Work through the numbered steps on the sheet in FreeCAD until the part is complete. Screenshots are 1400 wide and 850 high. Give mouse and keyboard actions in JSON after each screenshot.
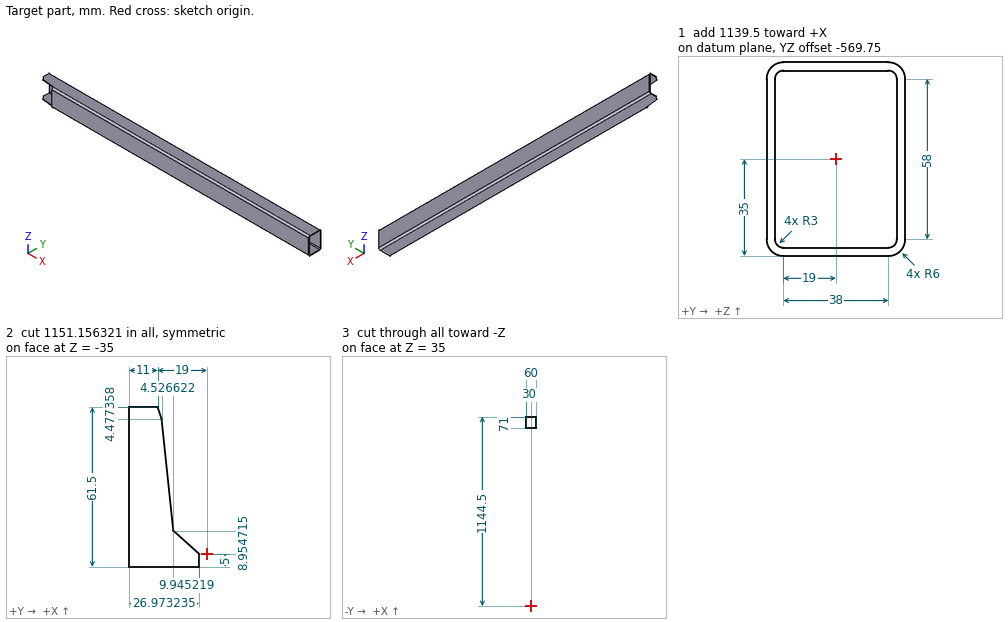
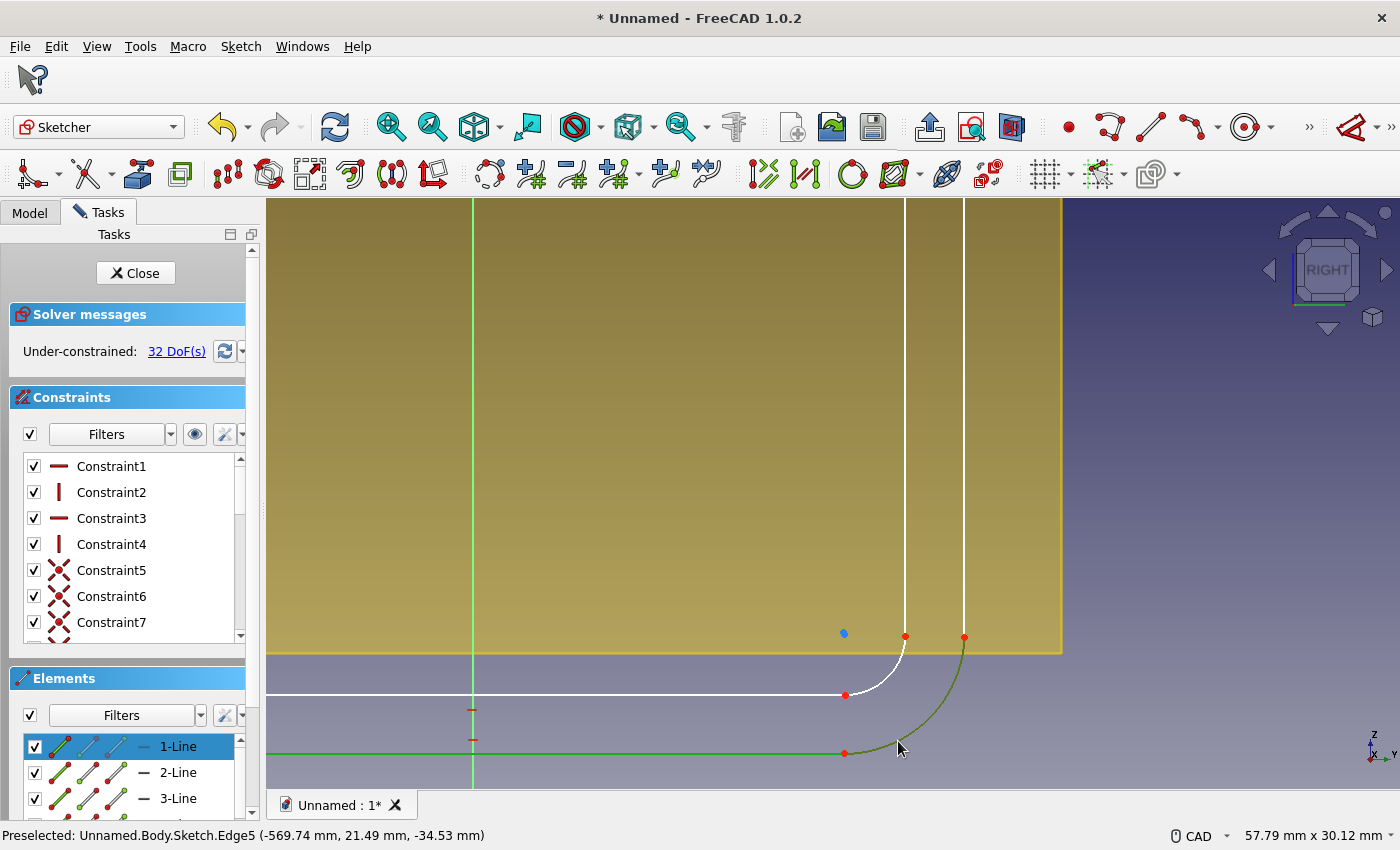
{"action": "key", "text": "t"}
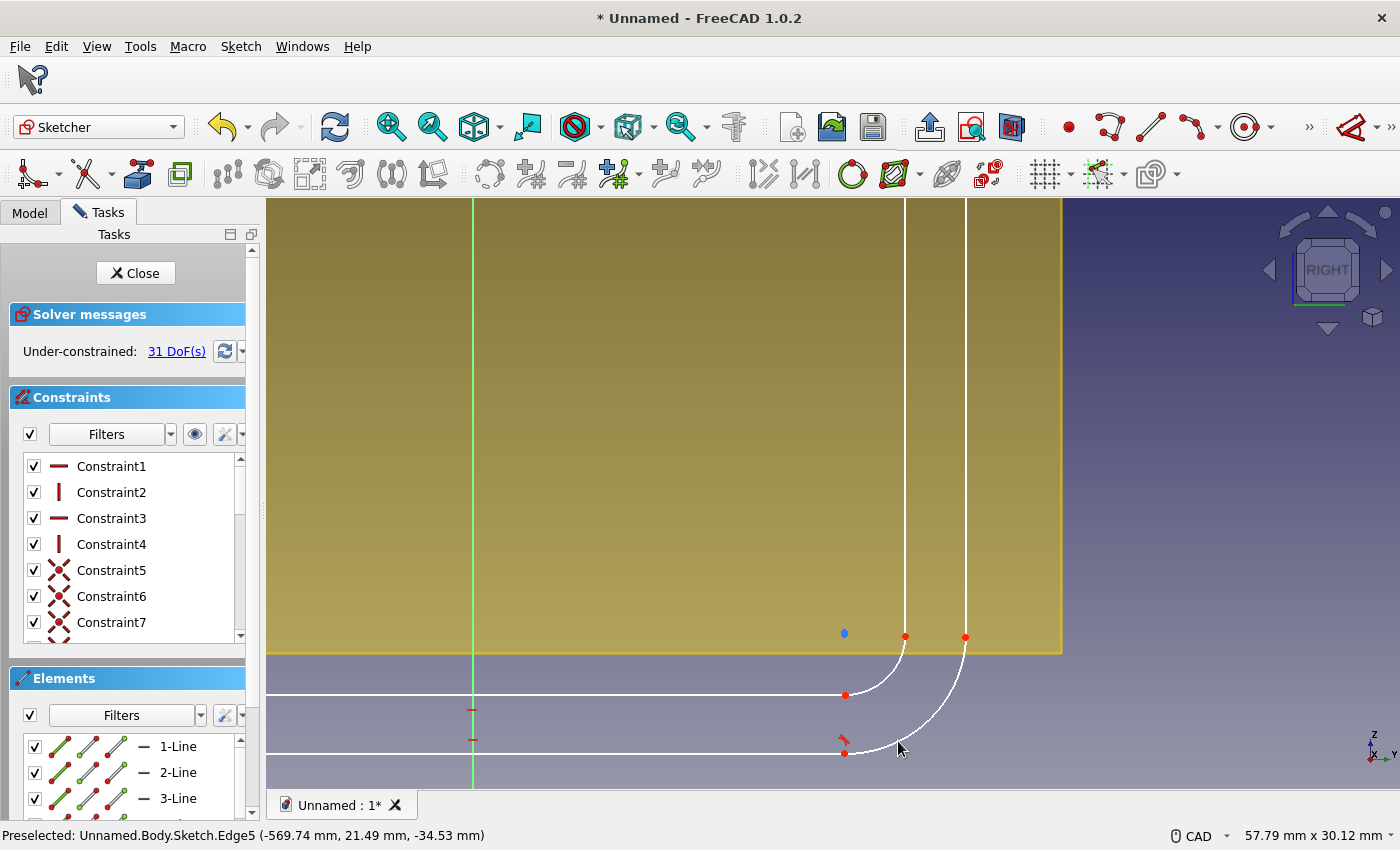
{"action": "left_click", "coordinate": [324, 754]}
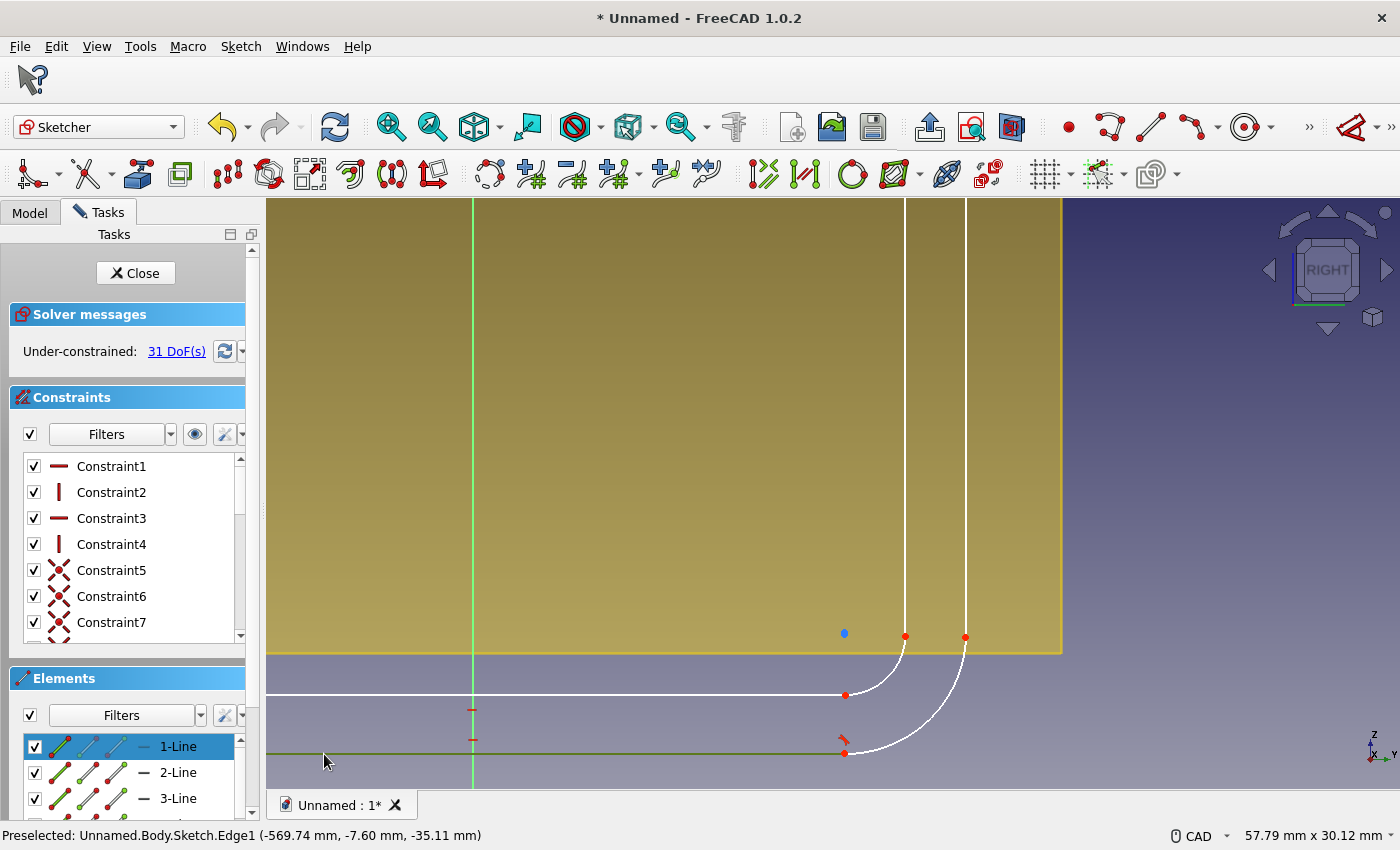
{"action": "scroll", "coordinate": [890, 678], "scroll_direction": "down", "scroll_amount": 6}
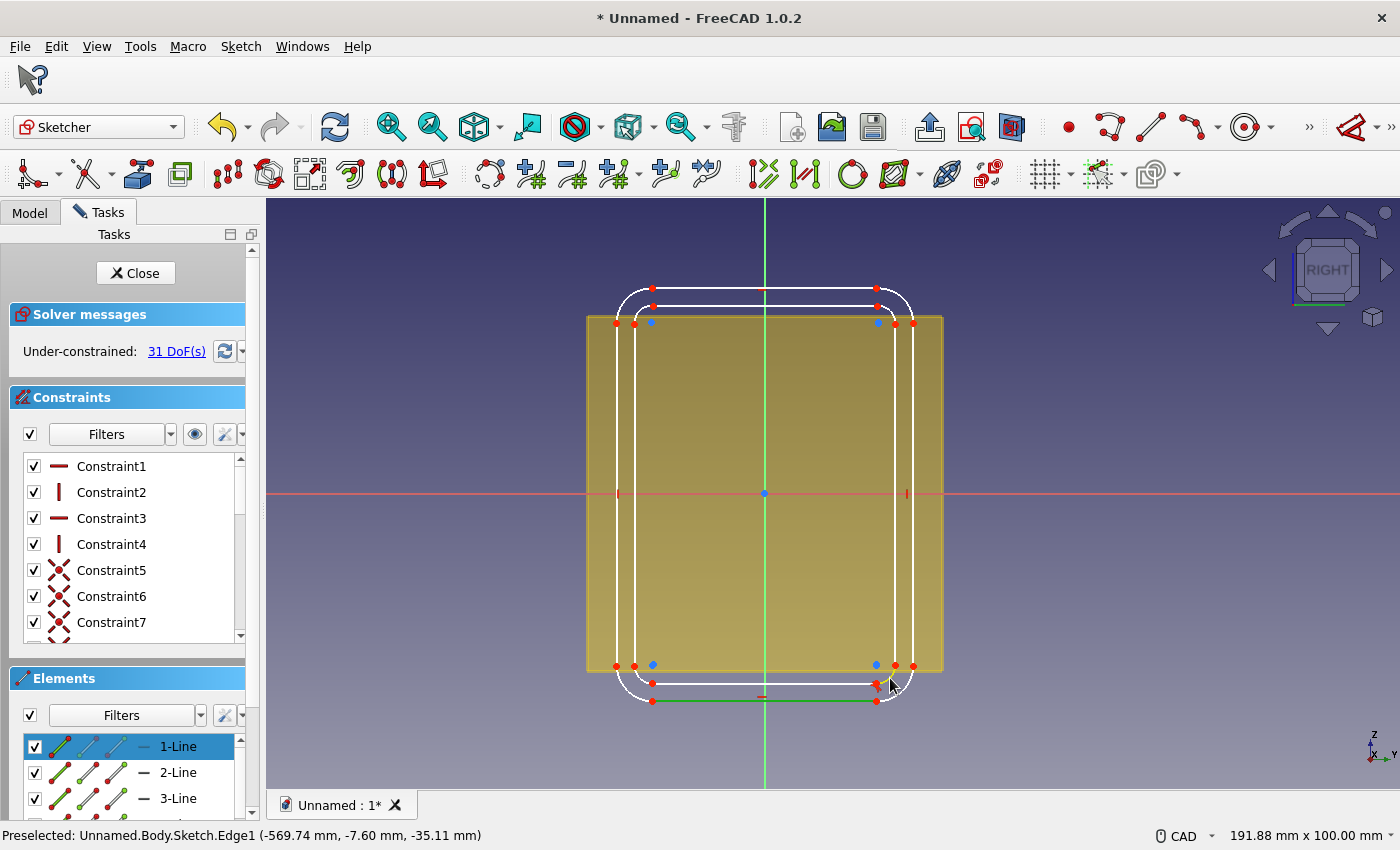
{"action": "left_click", "coordinate": [621, 682]}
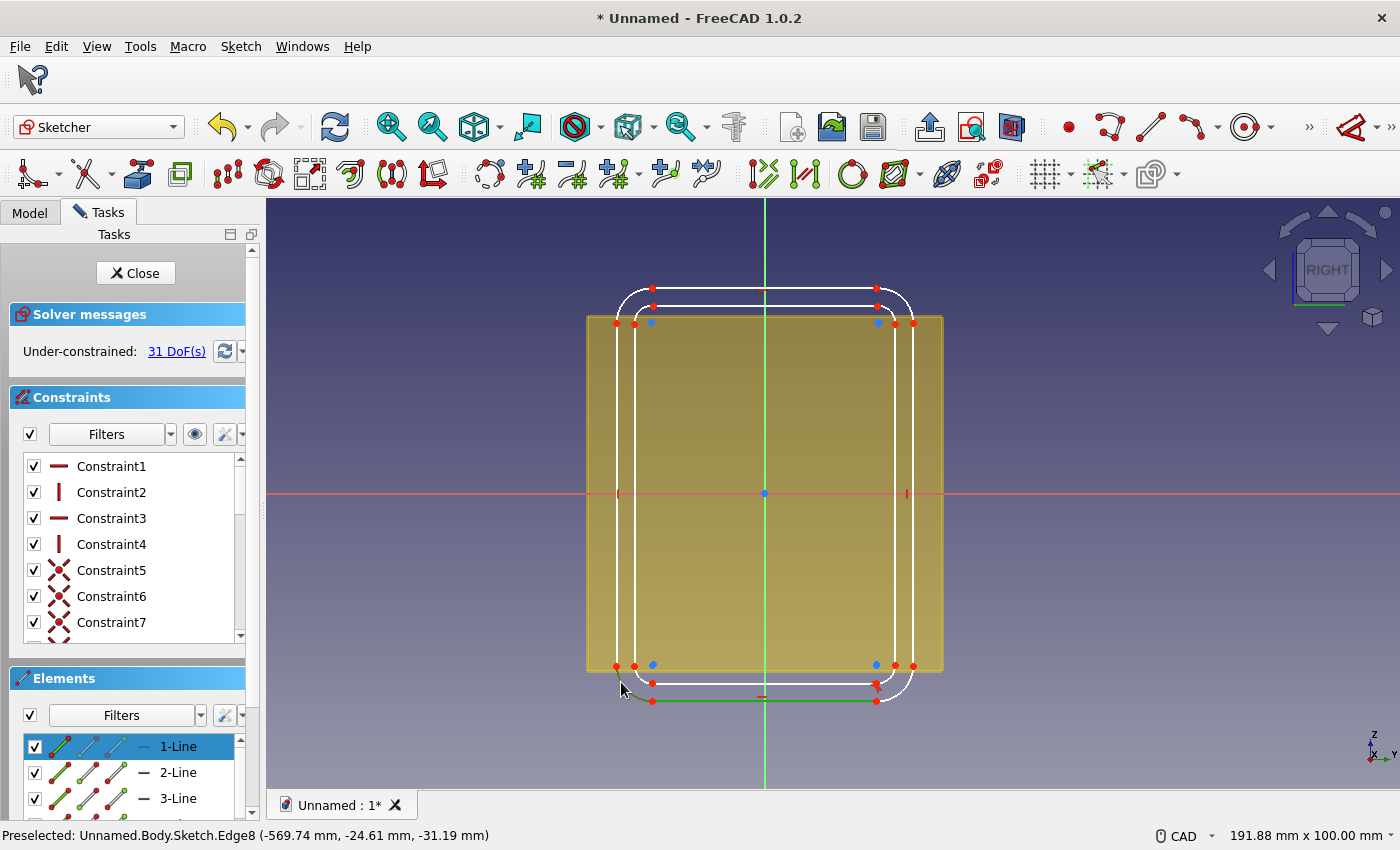
{"action": "key", "text": "t"}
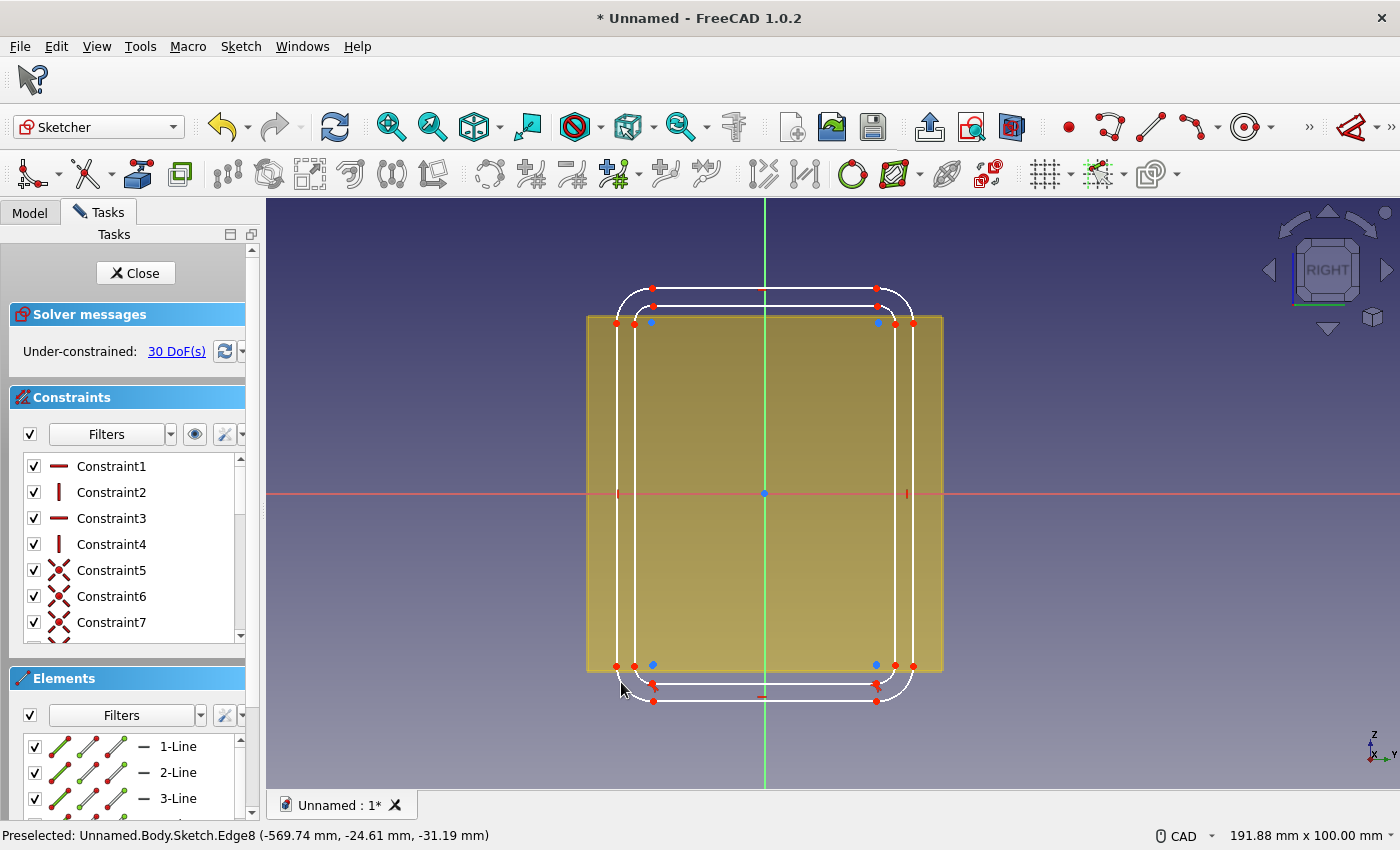
{"action": "left_click", "coordinate": [913, 564]}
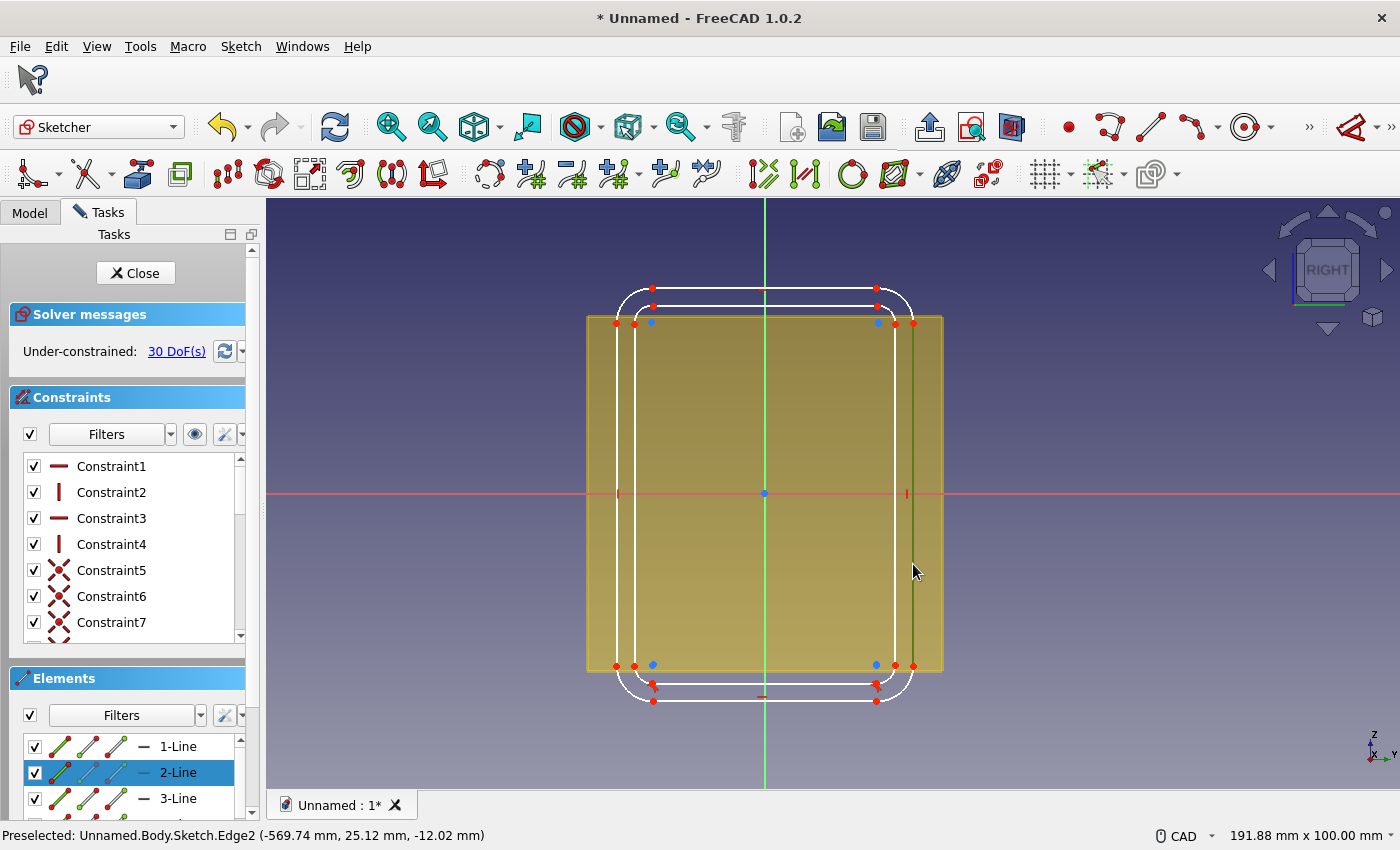
{"action": "left_click", "coordinate": [893, 698]}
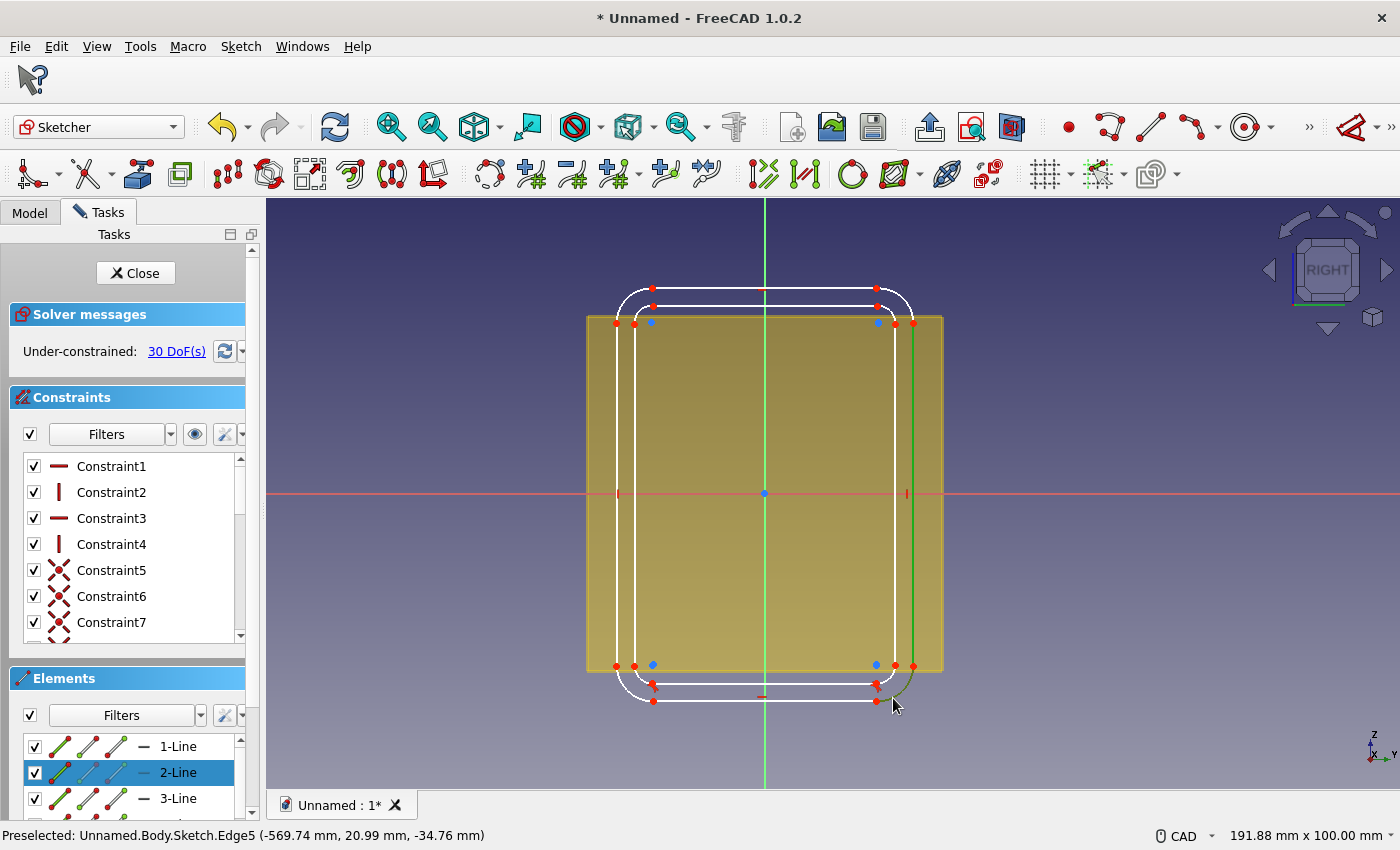
{"action": "key", "text": "t"}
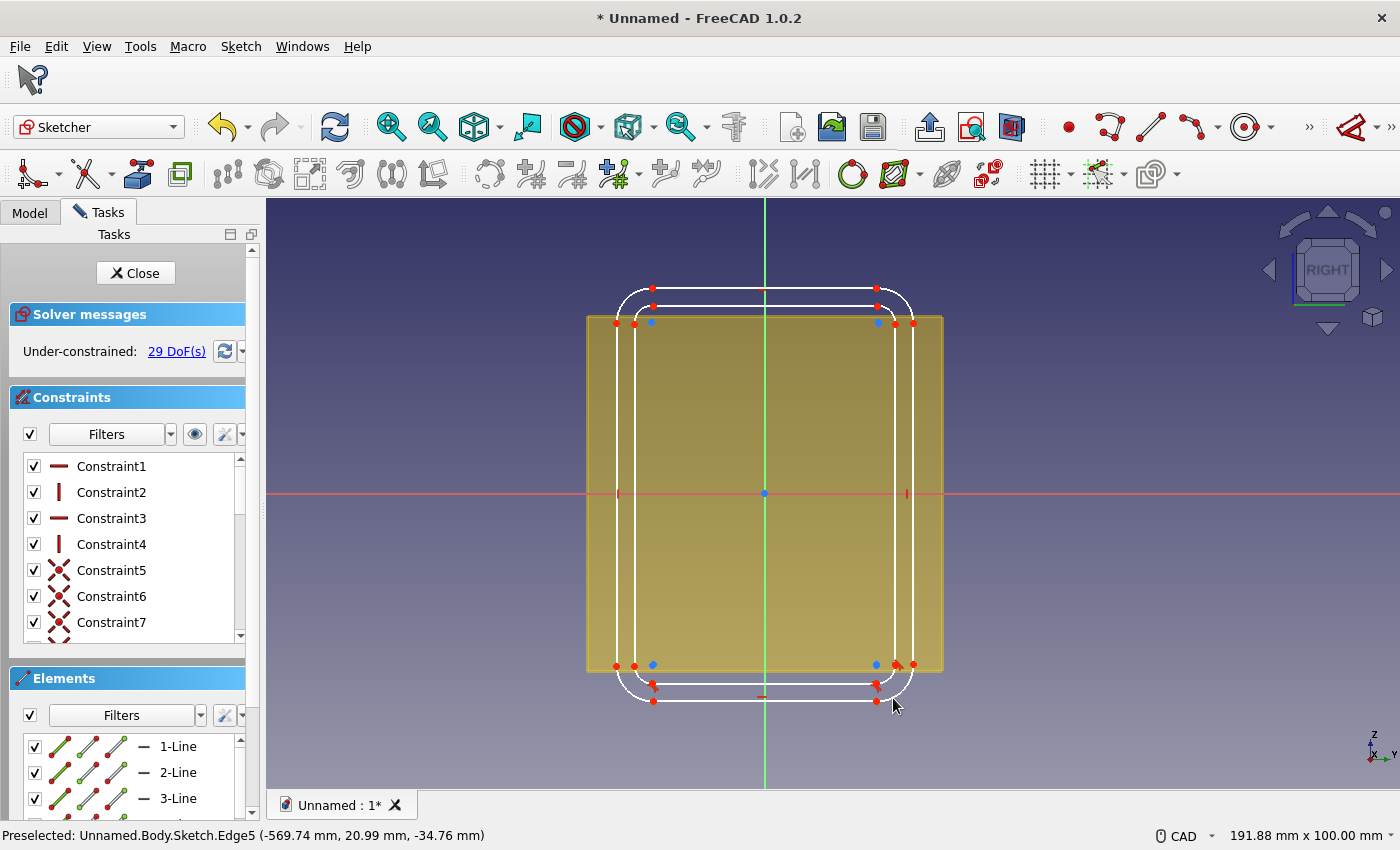
{"action": "left_click", "coordinate": [913, 563]}